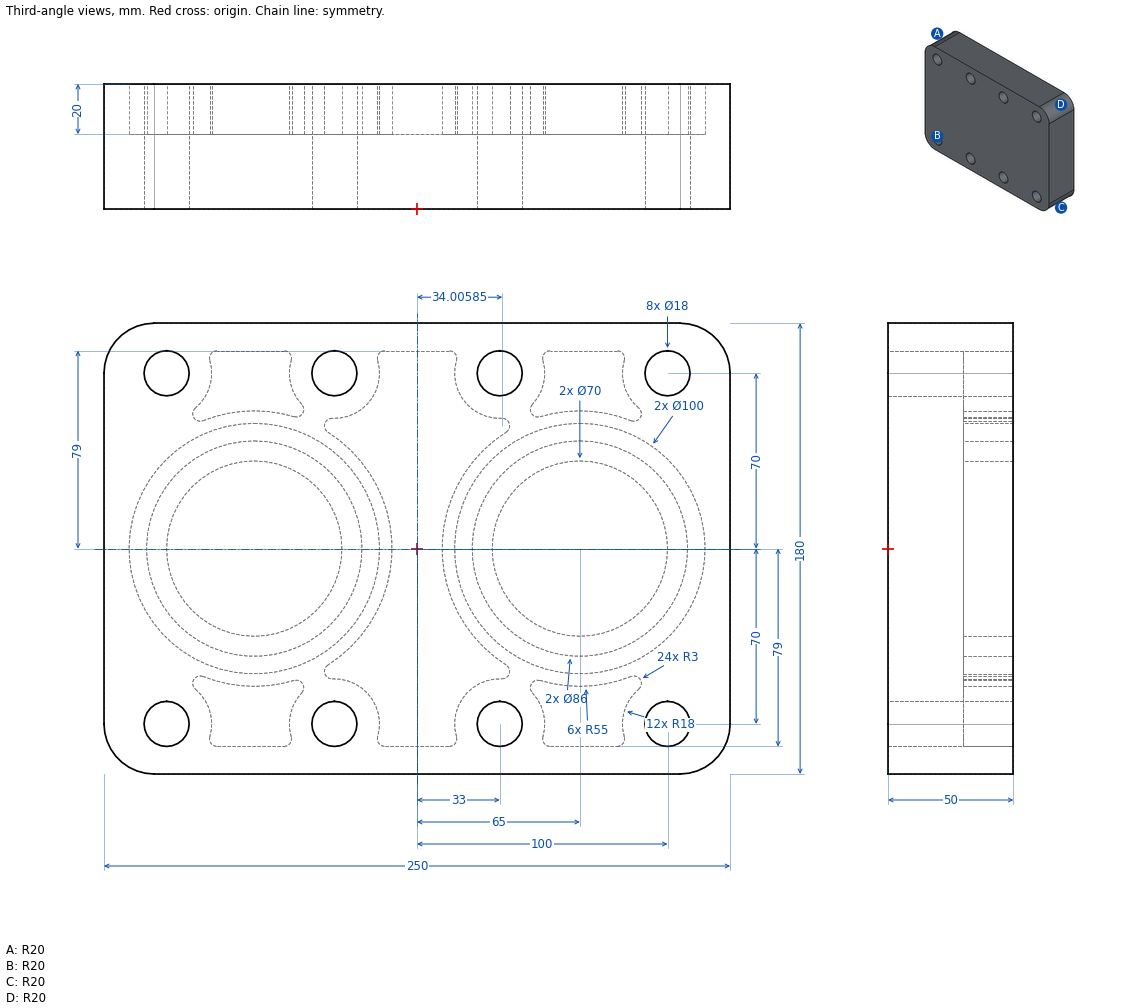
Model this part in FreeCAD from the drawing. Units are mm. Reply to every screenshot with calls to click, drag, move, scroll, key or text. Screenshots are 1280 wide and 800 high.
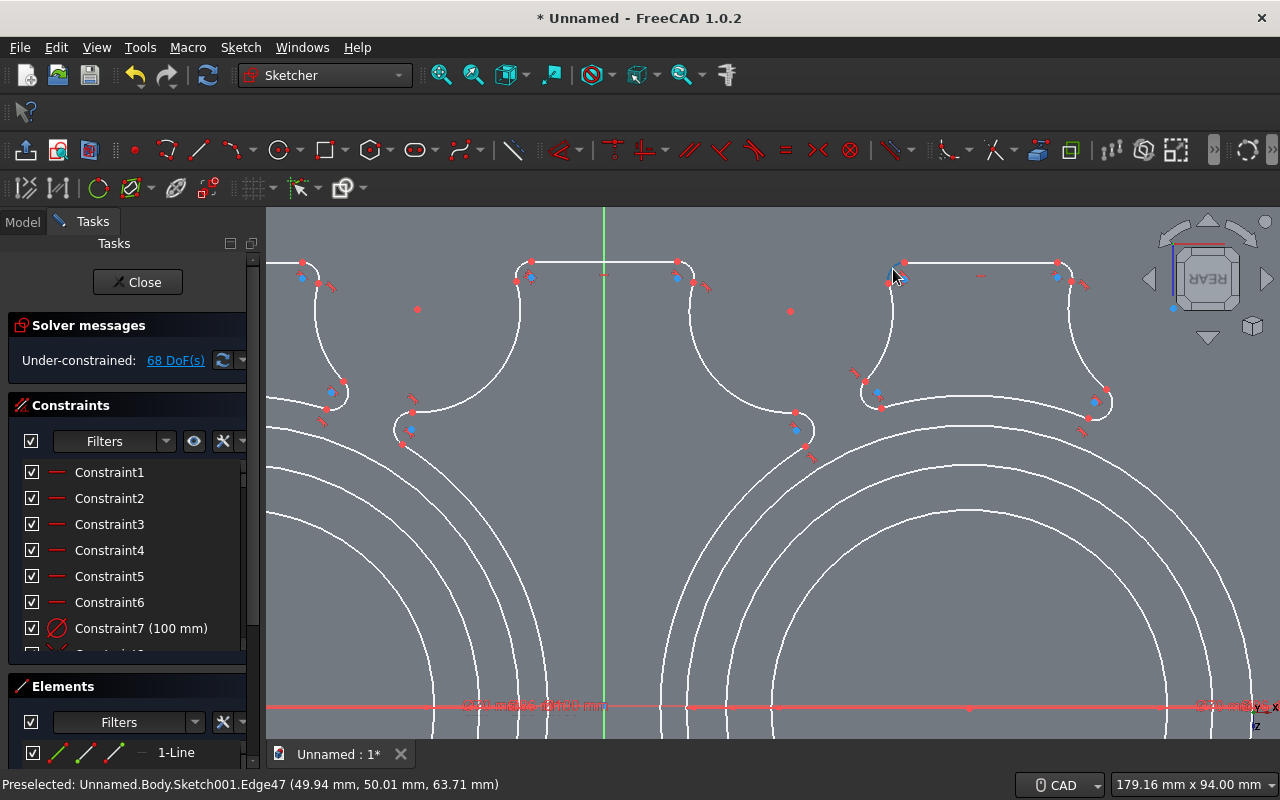
click(892, 269)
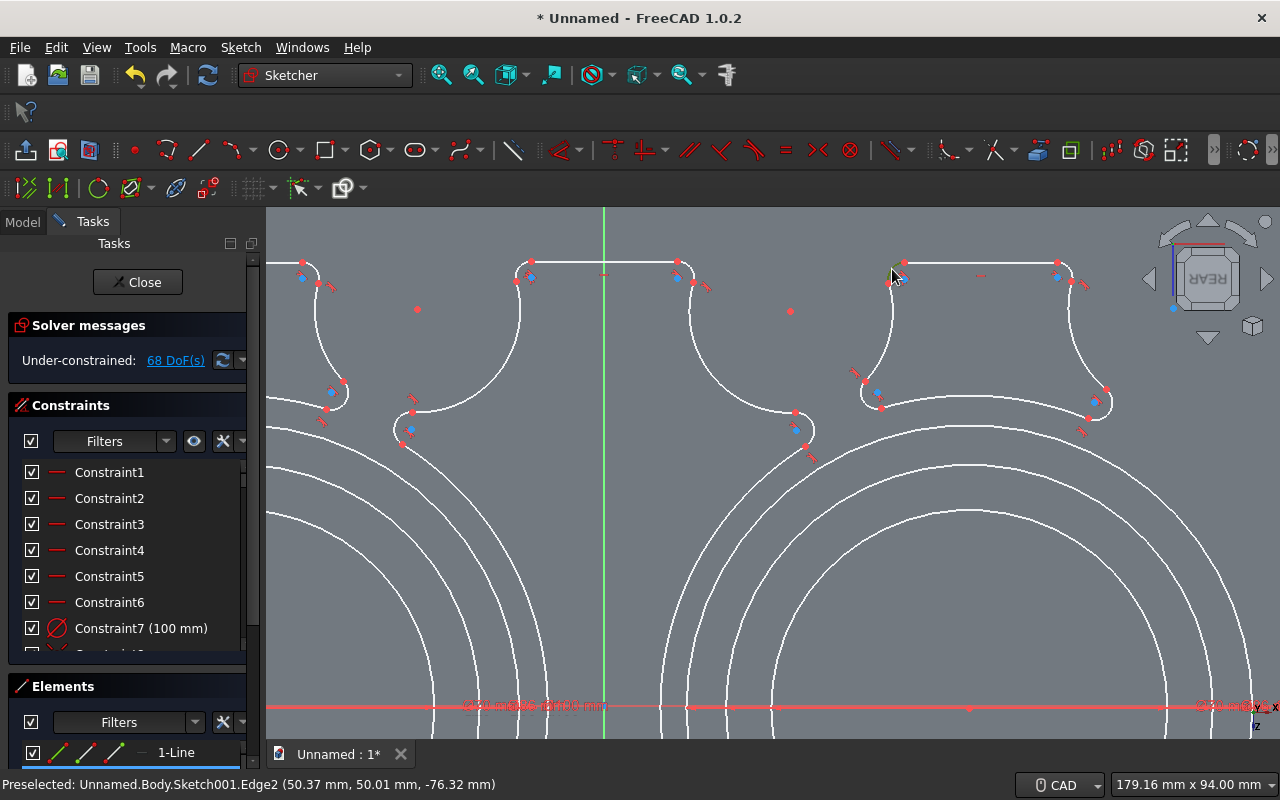
click(861, 393)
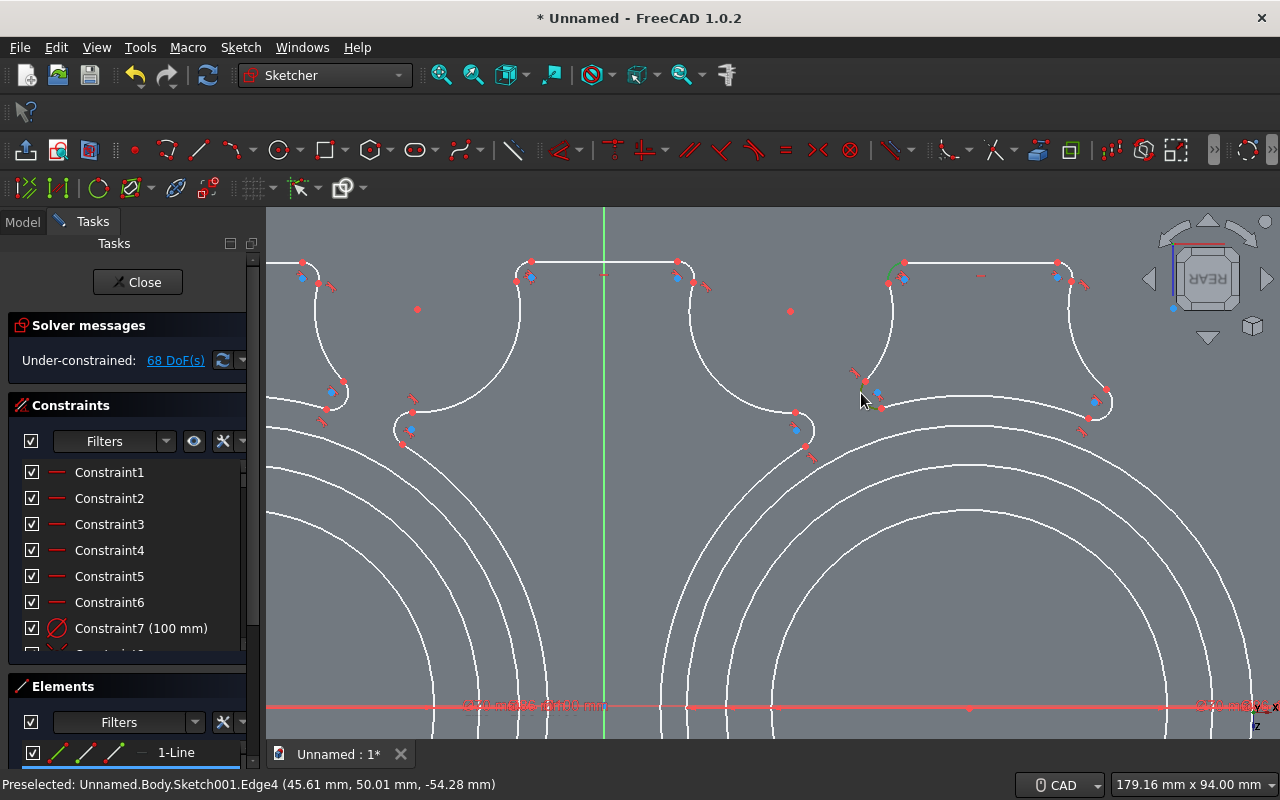
click(1103, 418)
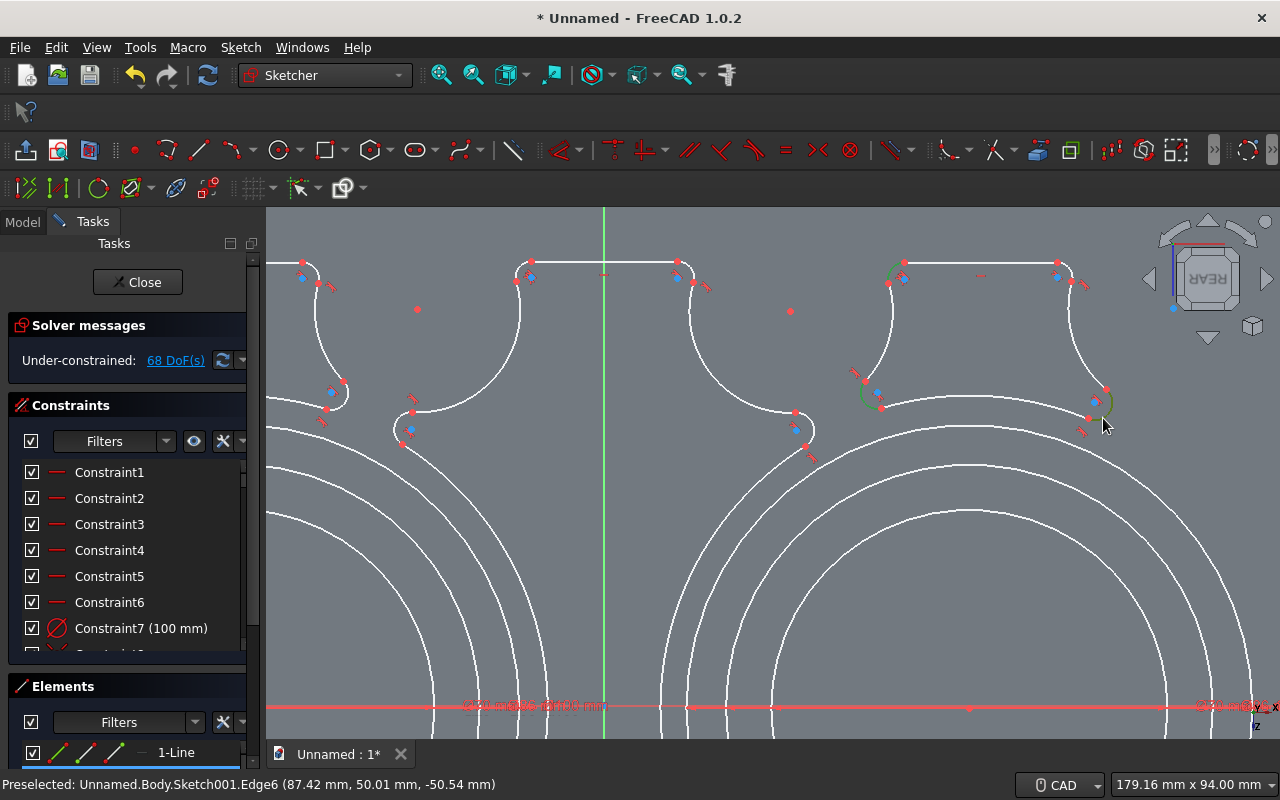
click(1069, 268)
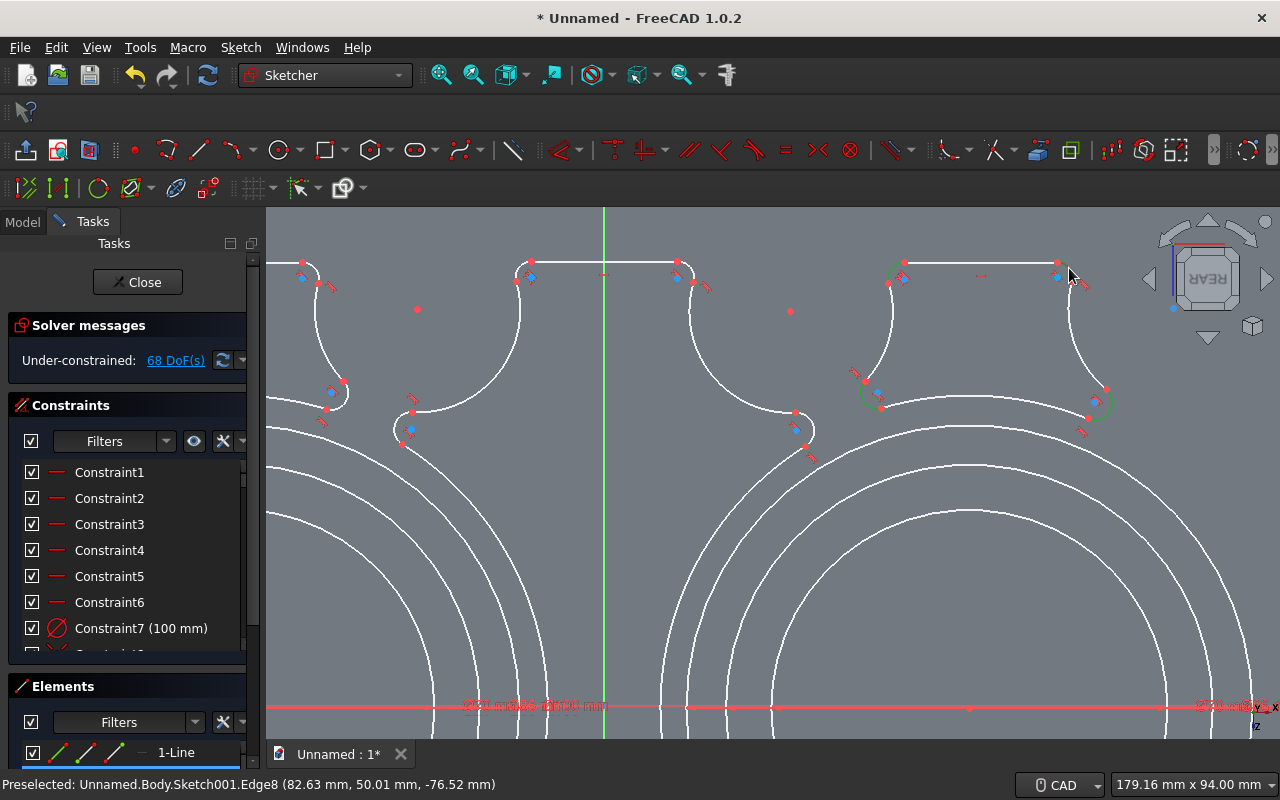
scroll(763, 337, down, 5)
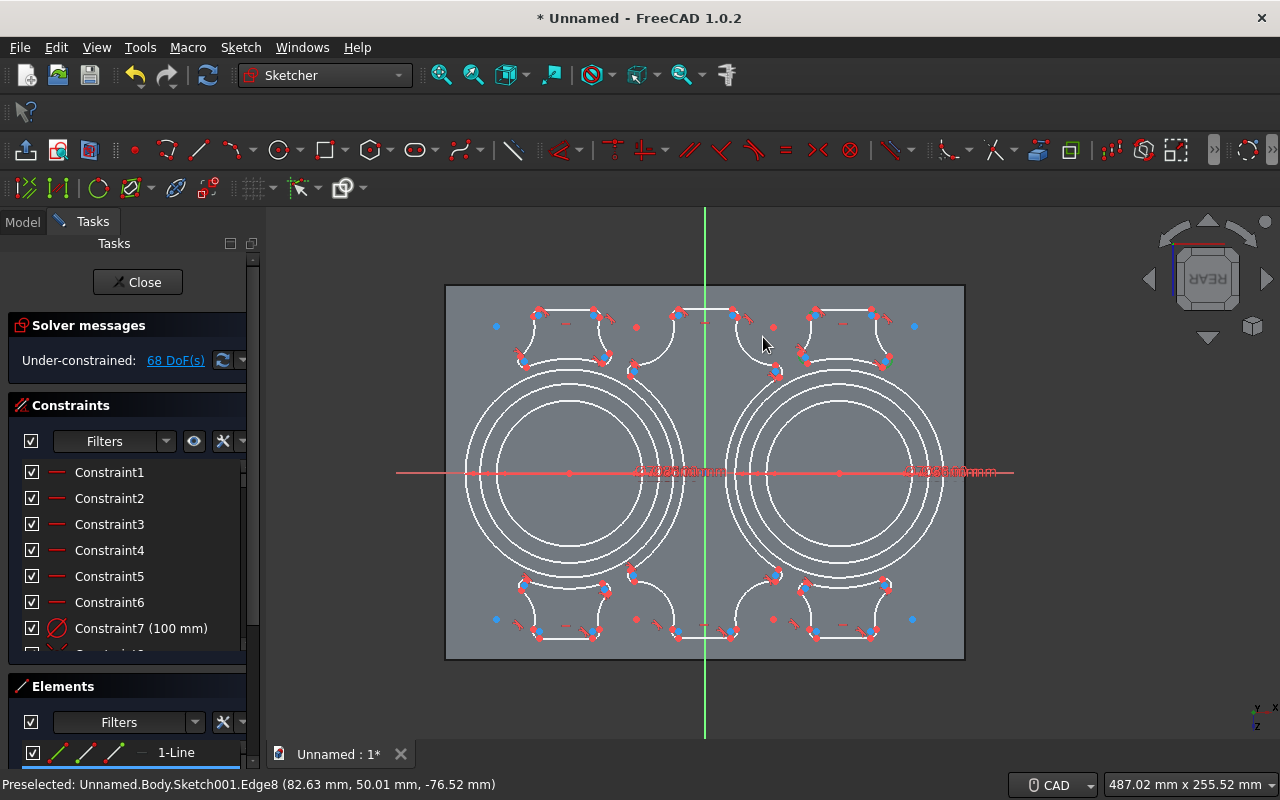
scroll(734, 637, up, 7)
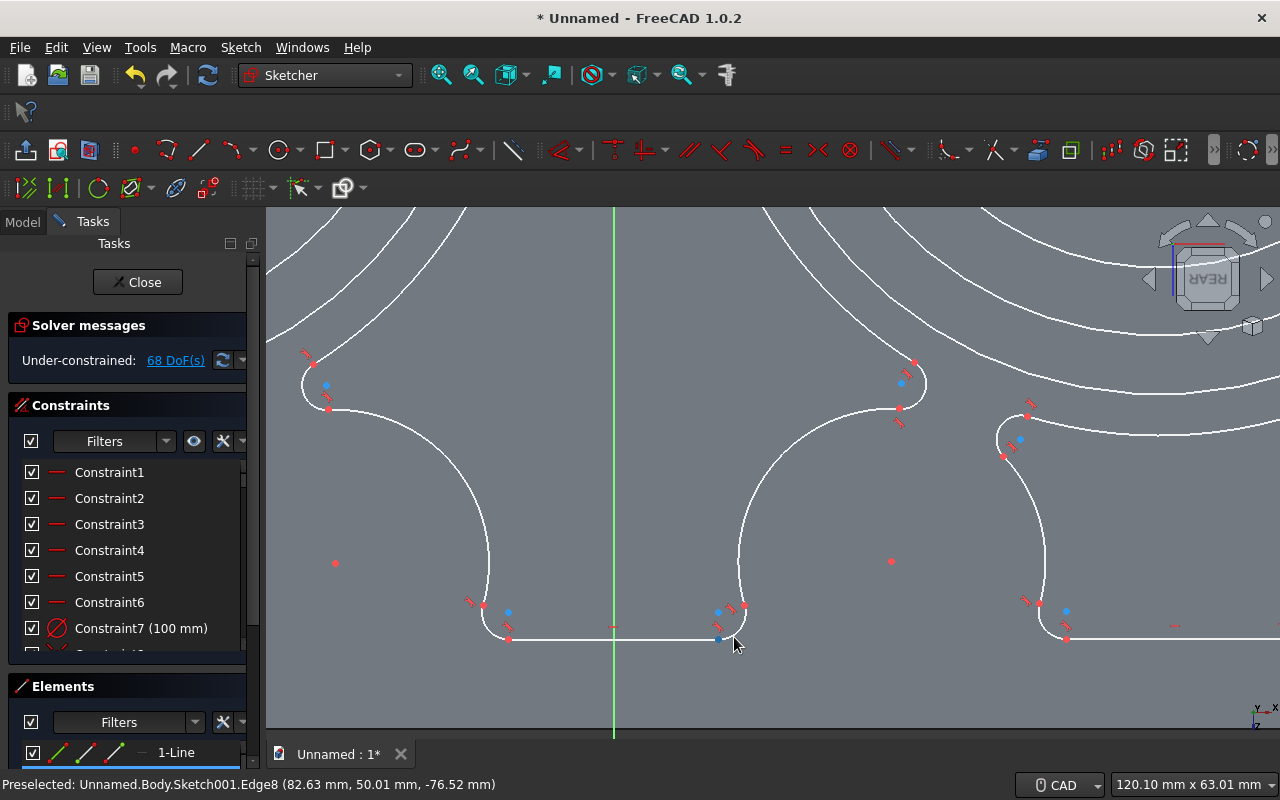
click(733, 635)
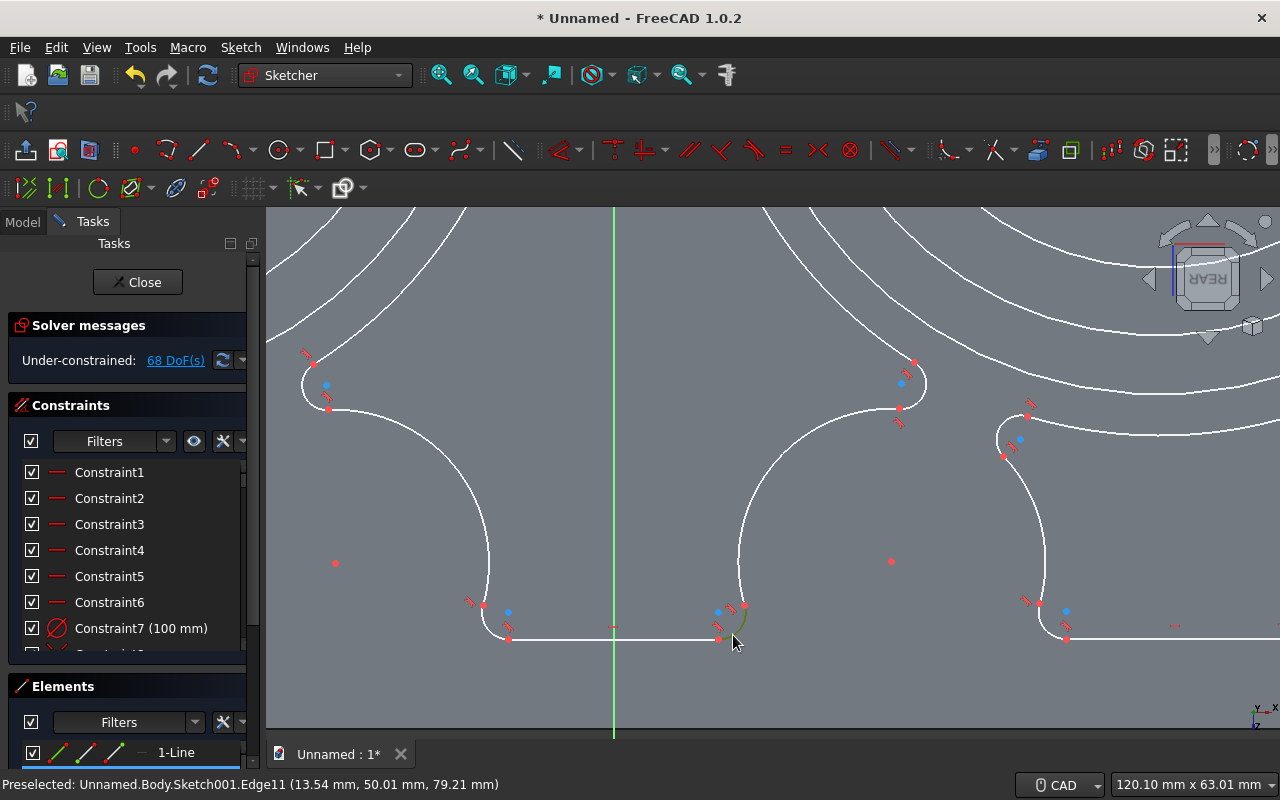
click(918, 402)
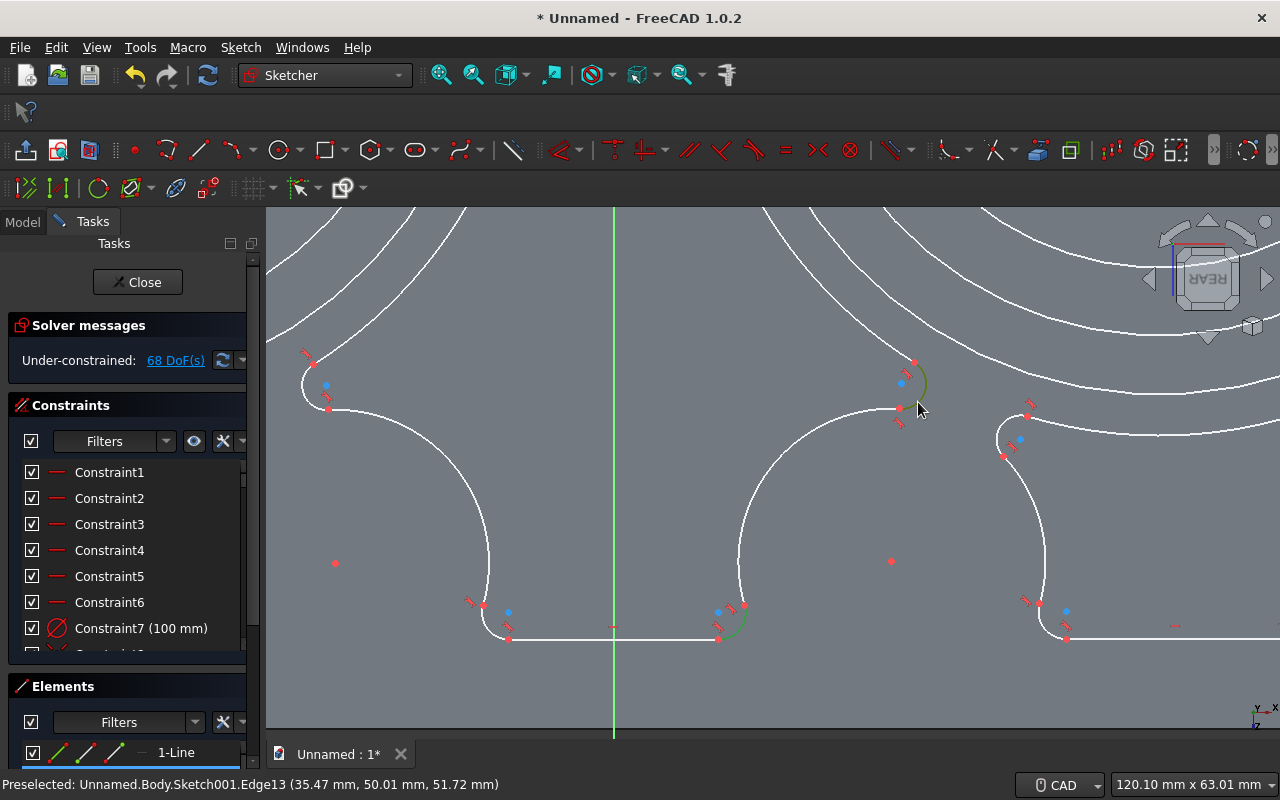
scroll(734, 638, down, 7)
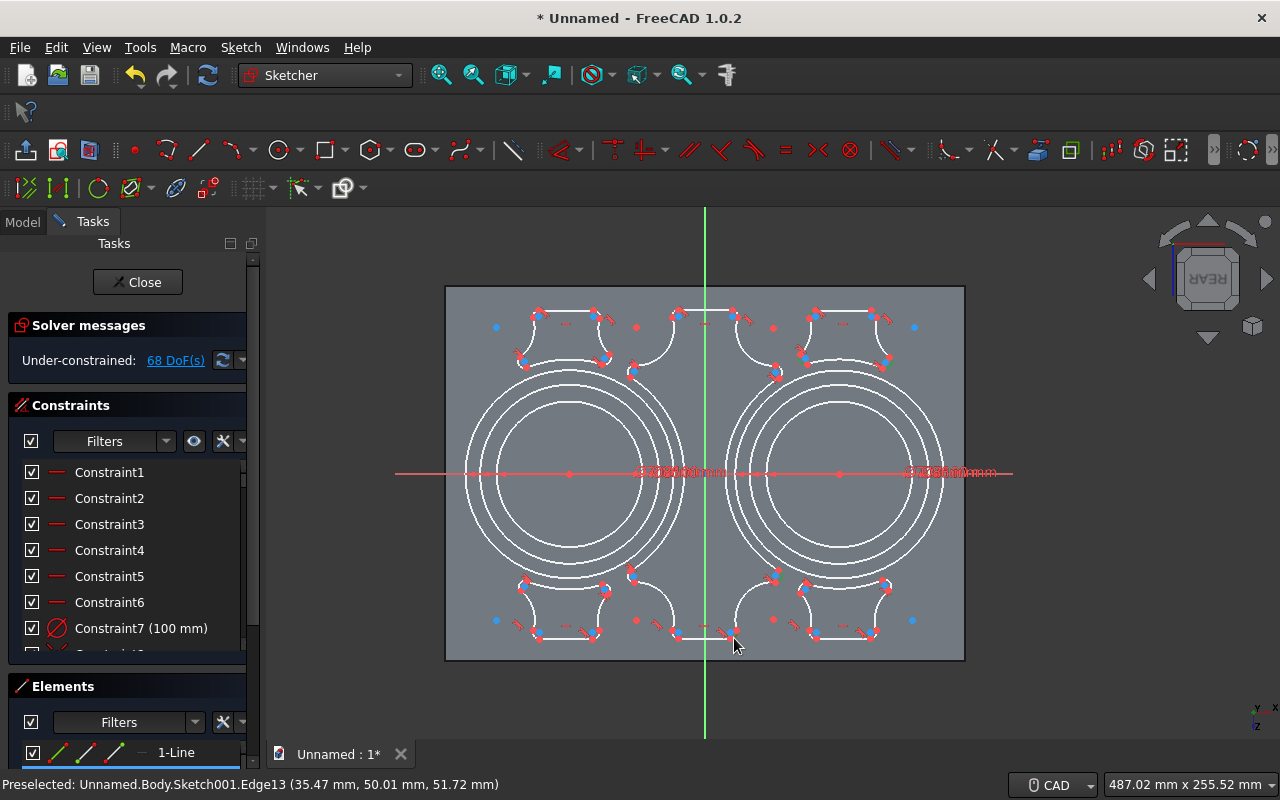
scroll(782, 374, up, 5)